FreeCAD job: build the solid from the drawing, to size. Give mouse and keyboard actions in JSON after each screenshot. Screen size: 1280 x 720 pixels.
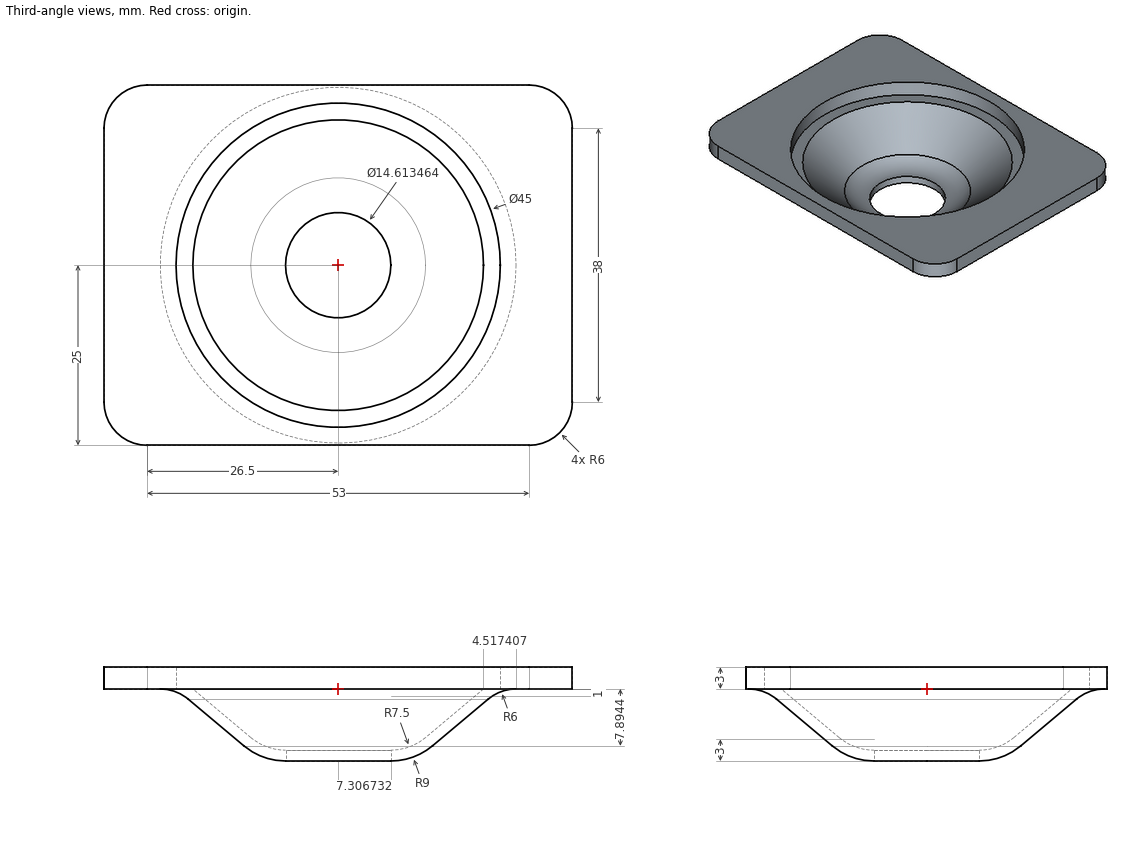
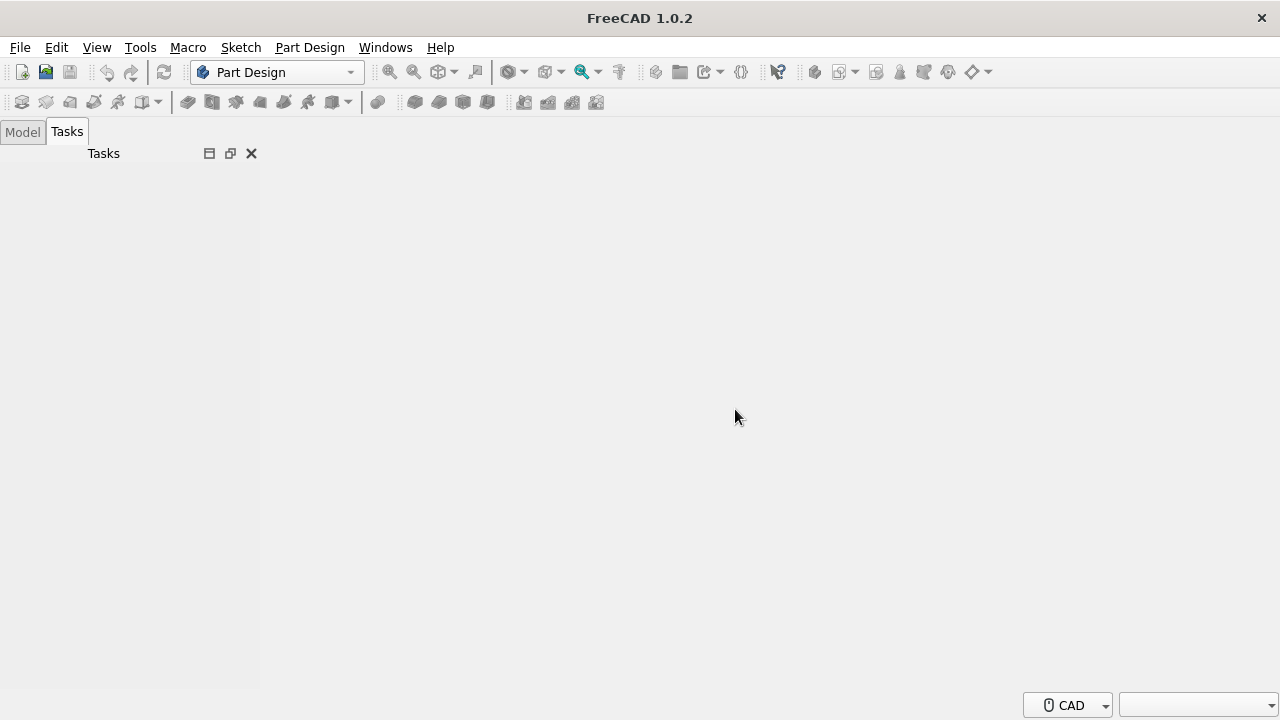
{"action": "key", "text": "ctrl+n"}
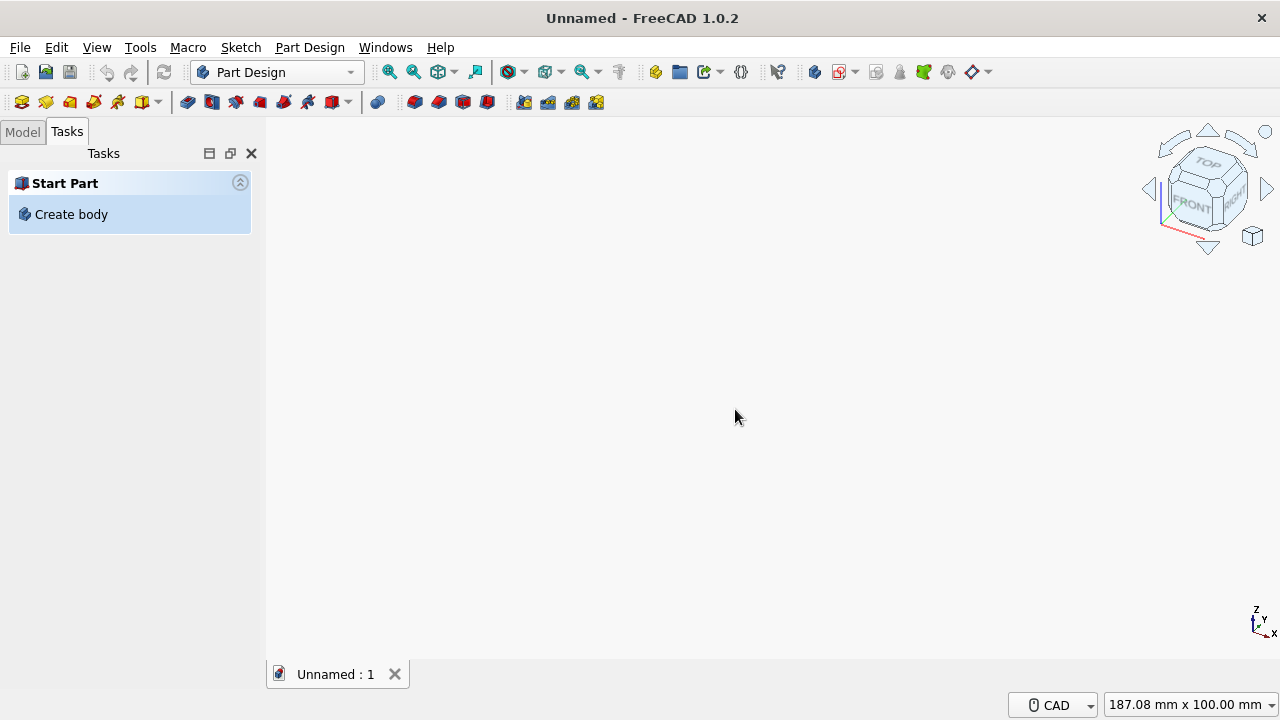
{"action": "left_click", "coordinate": [840, 72]}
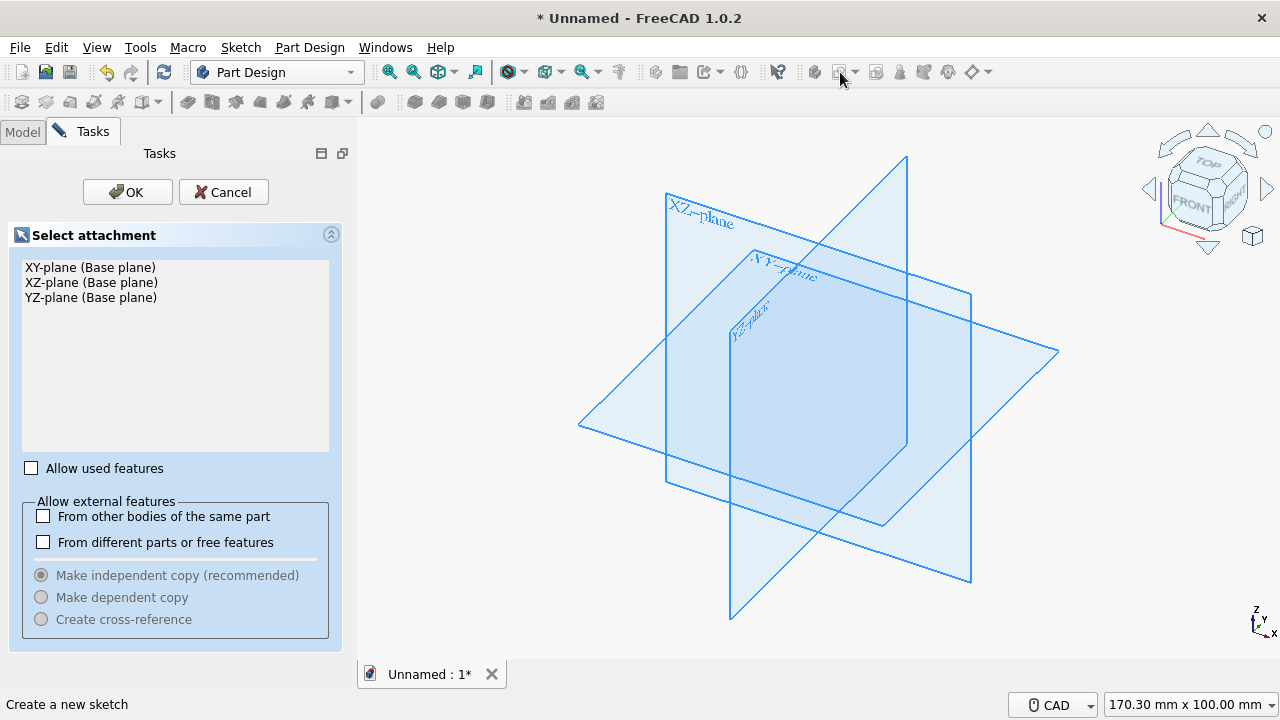
{"action": "left_click", "coordinate": [82, 268]}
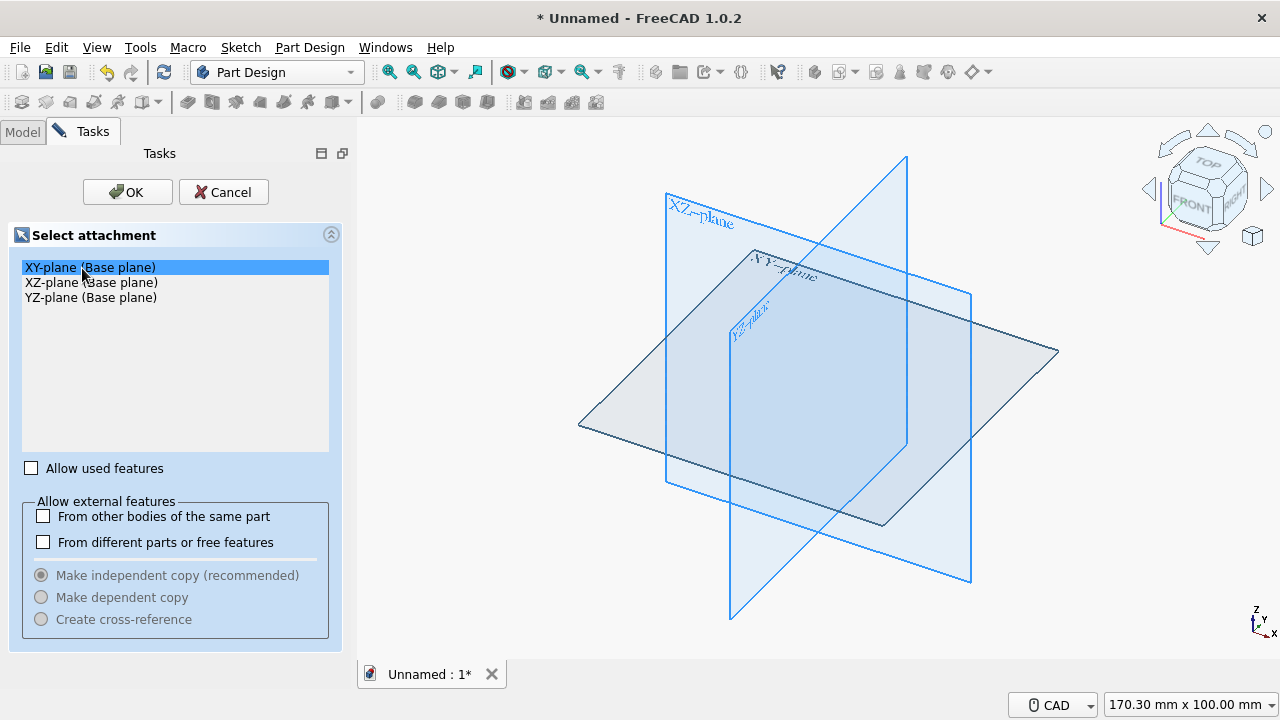
{"action": "left_click", "coordinate": [128, 192]}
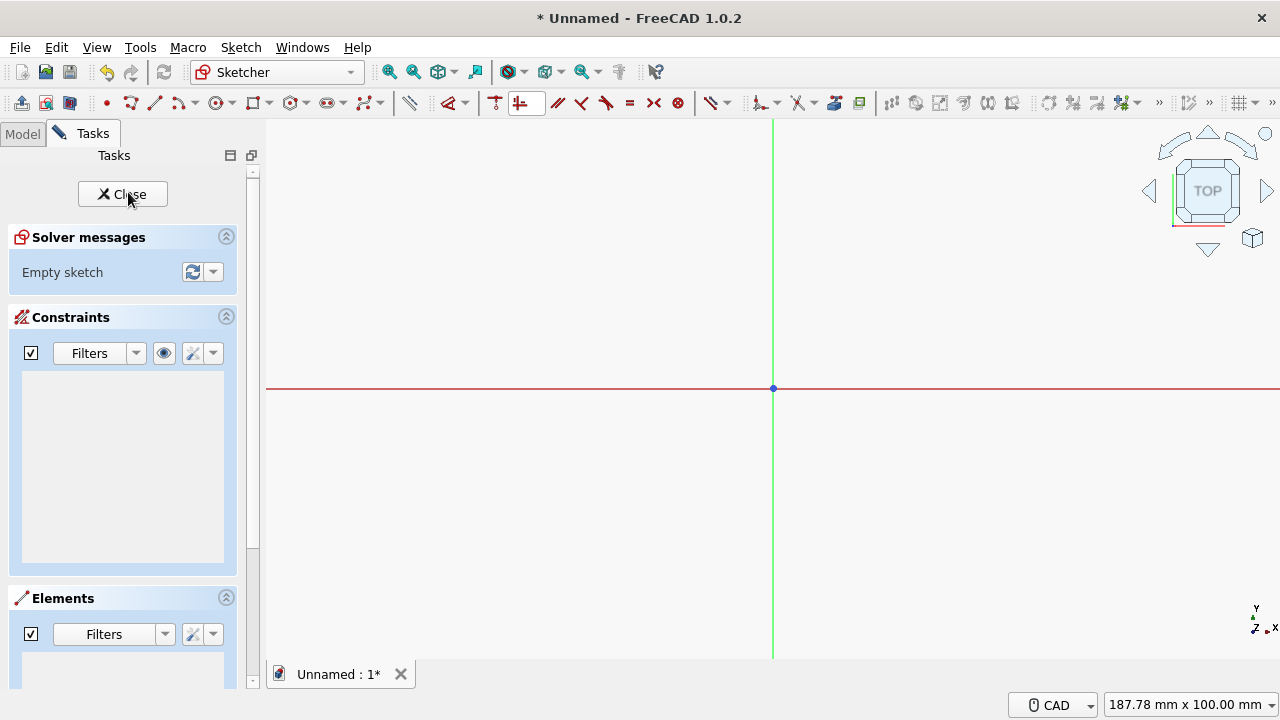
{"action": "key", "text": "g l"}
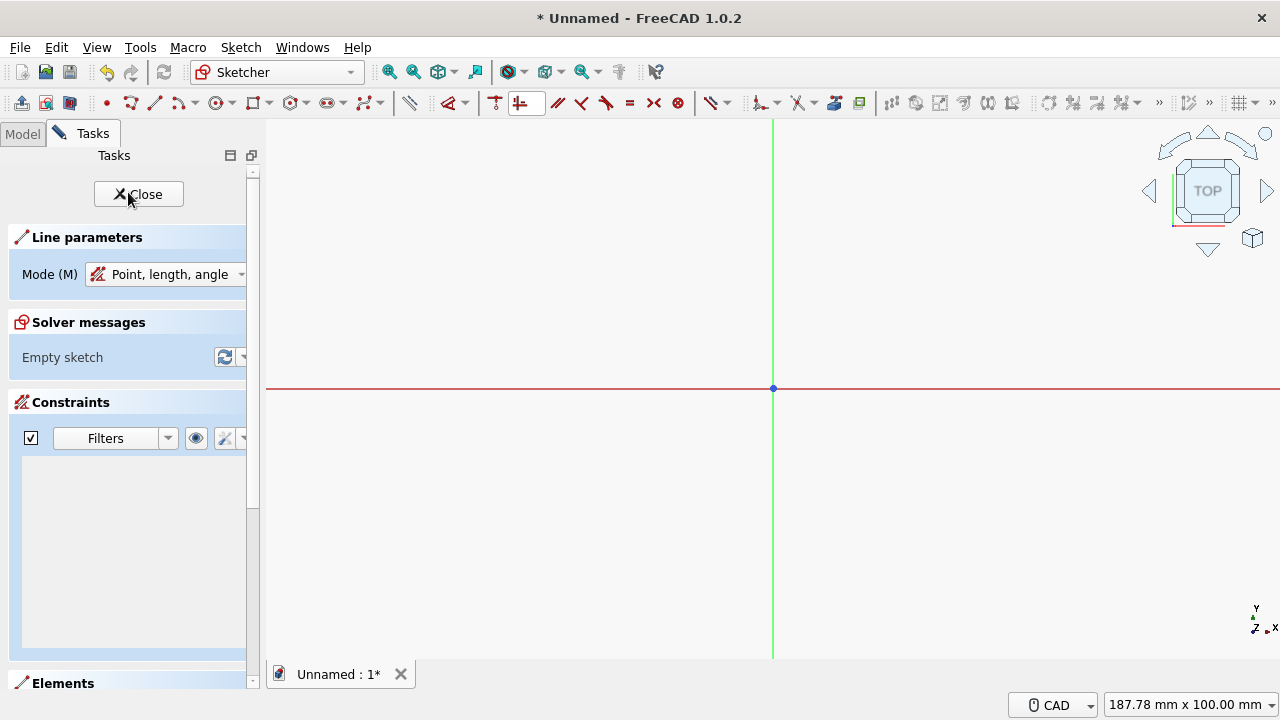
{"action": "left_click", "coordinate": [630, 524]}
{"action": "left_click", "coordinate": [916, 524]}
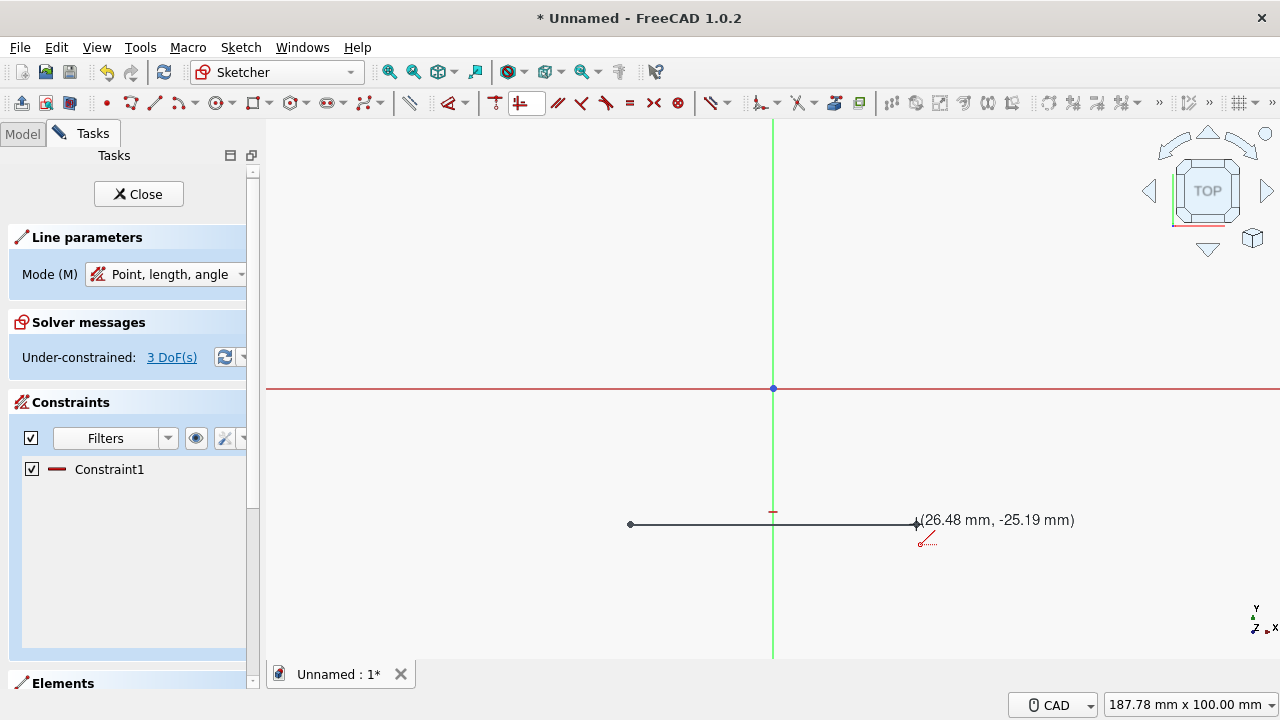
{"action": "left_click", "coordinate": [948, 492]}
{"action": "left_click", "coordinate": [948, 286]}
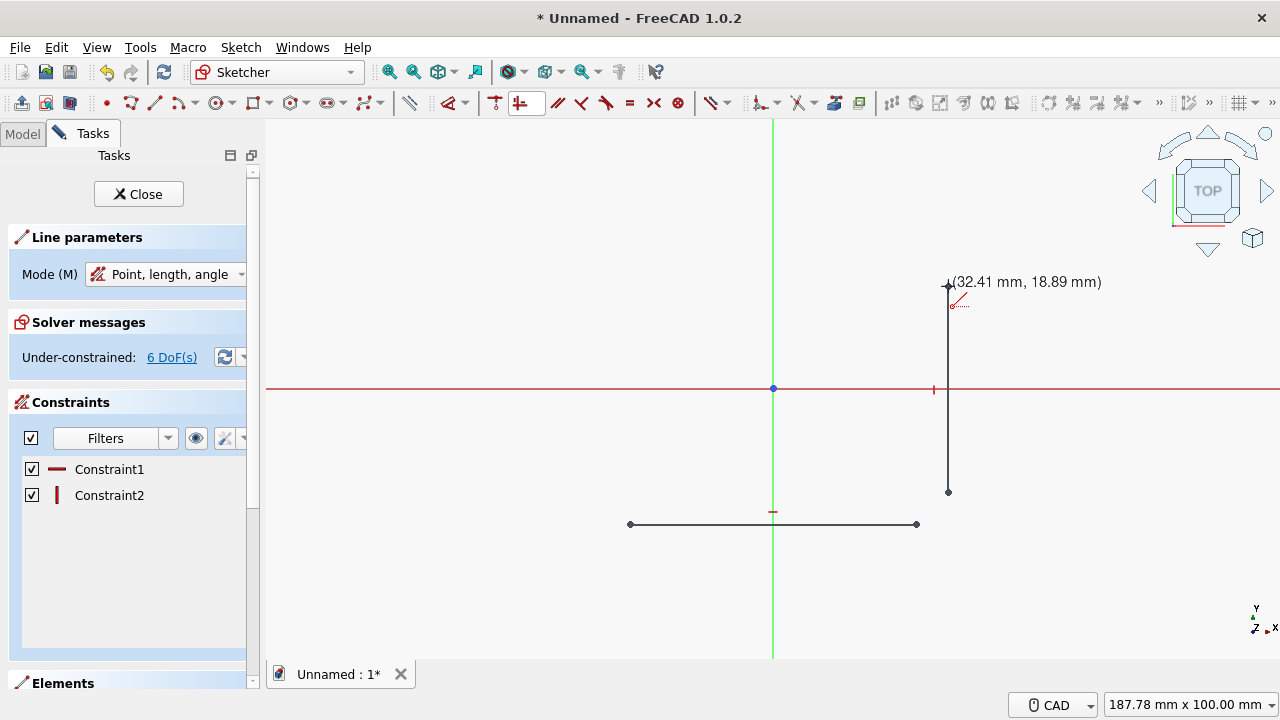
{"action": "left_click", "coordinate": [916, 254]}
{"action": "left_click", "coordinate": [630, 254]}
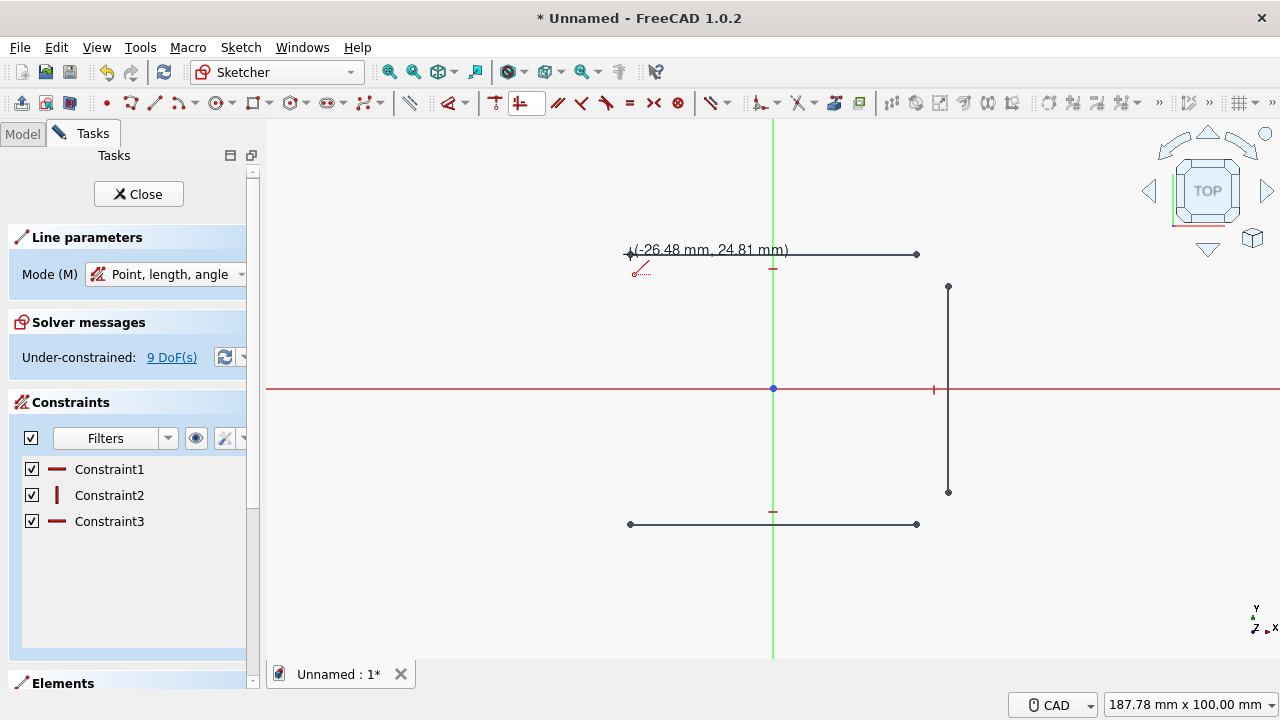
{"action": "left_click", "coordinate": [598, 286]}
{"action": "left_click", "coordinate": [598, 492]}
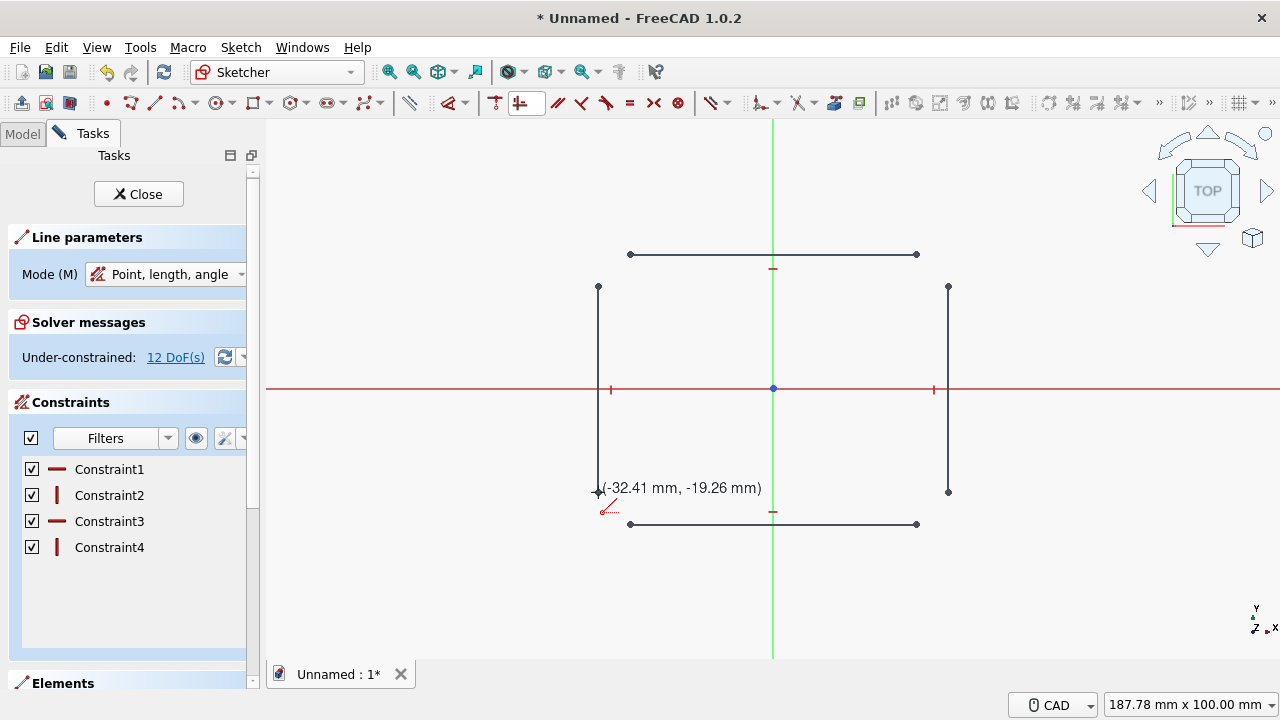
{"action": "key", "text": "g 3 a"}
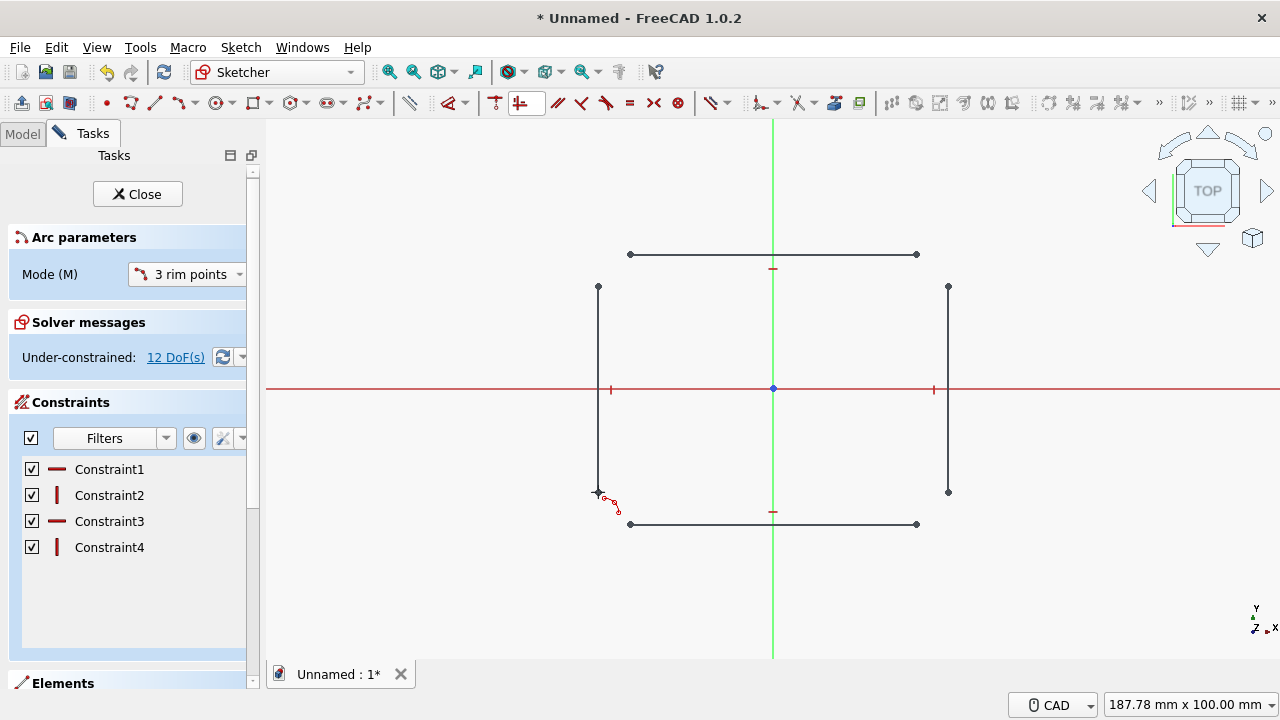
{"action": "left_click", "coordinate": [916, 525]}
{"action": "left_click", "coordinate": [948, 493]}